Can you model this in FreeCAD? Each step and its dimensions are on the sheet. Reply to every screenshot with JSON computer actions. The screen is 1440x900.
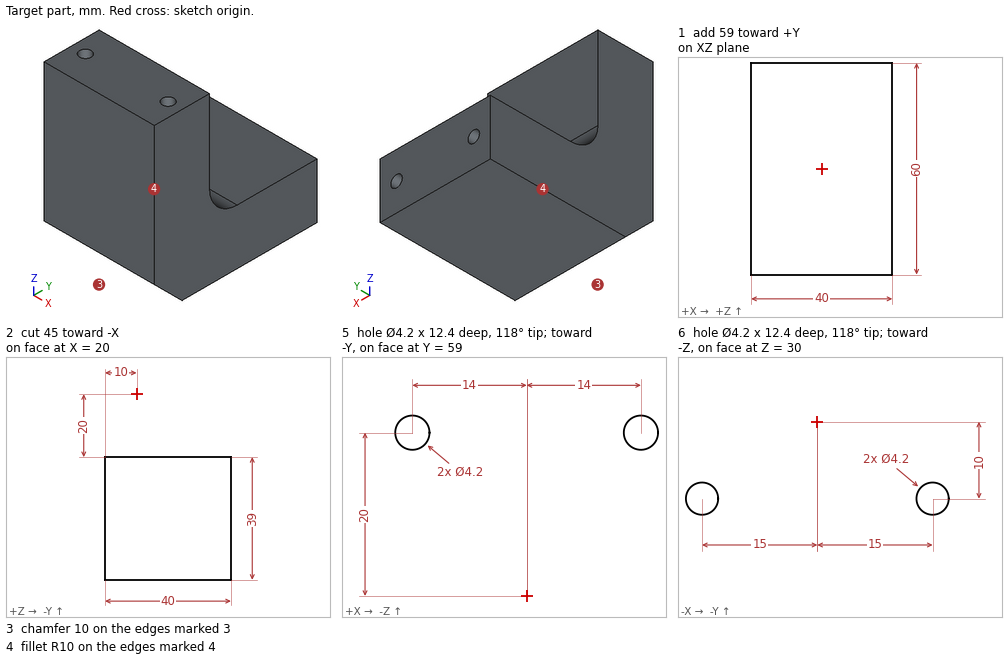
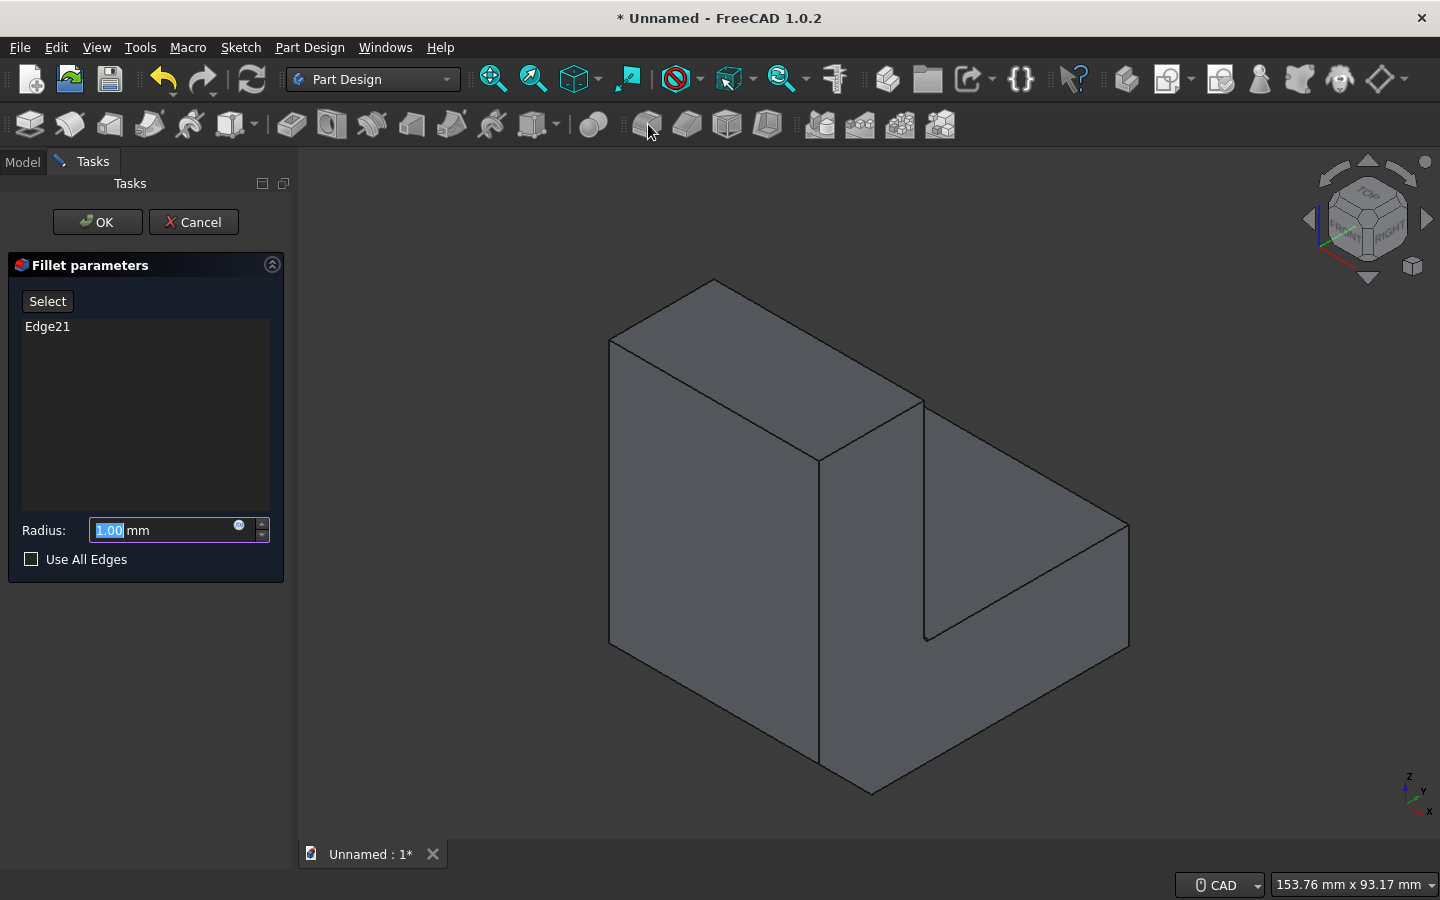
{"action": "type", "text": "10"}
{"action": "key", "text": "Tab"}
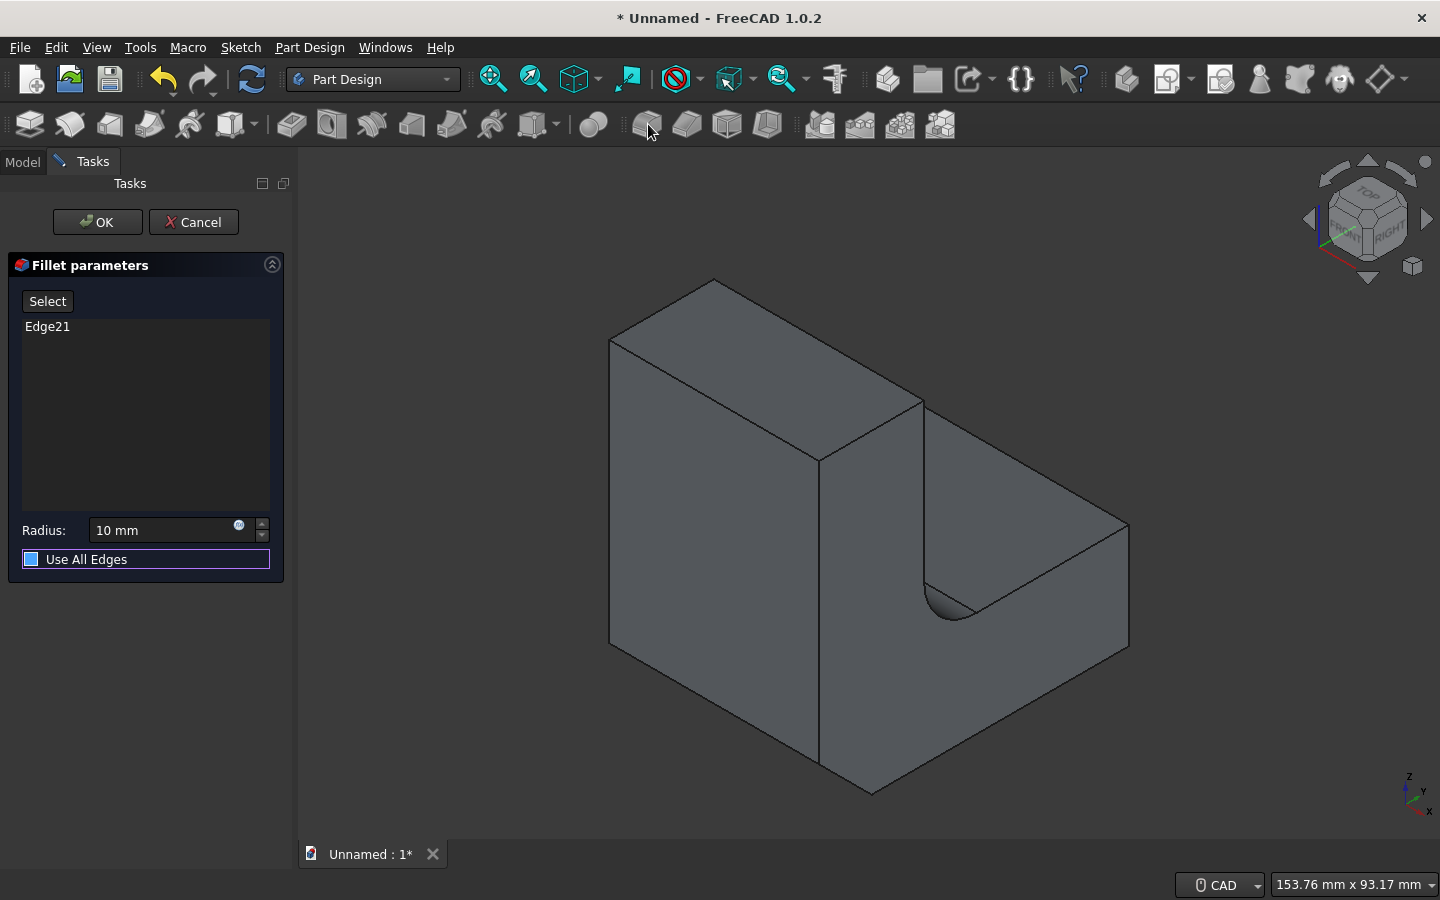
{"action": "left_click", "coordinate": [98, 222]}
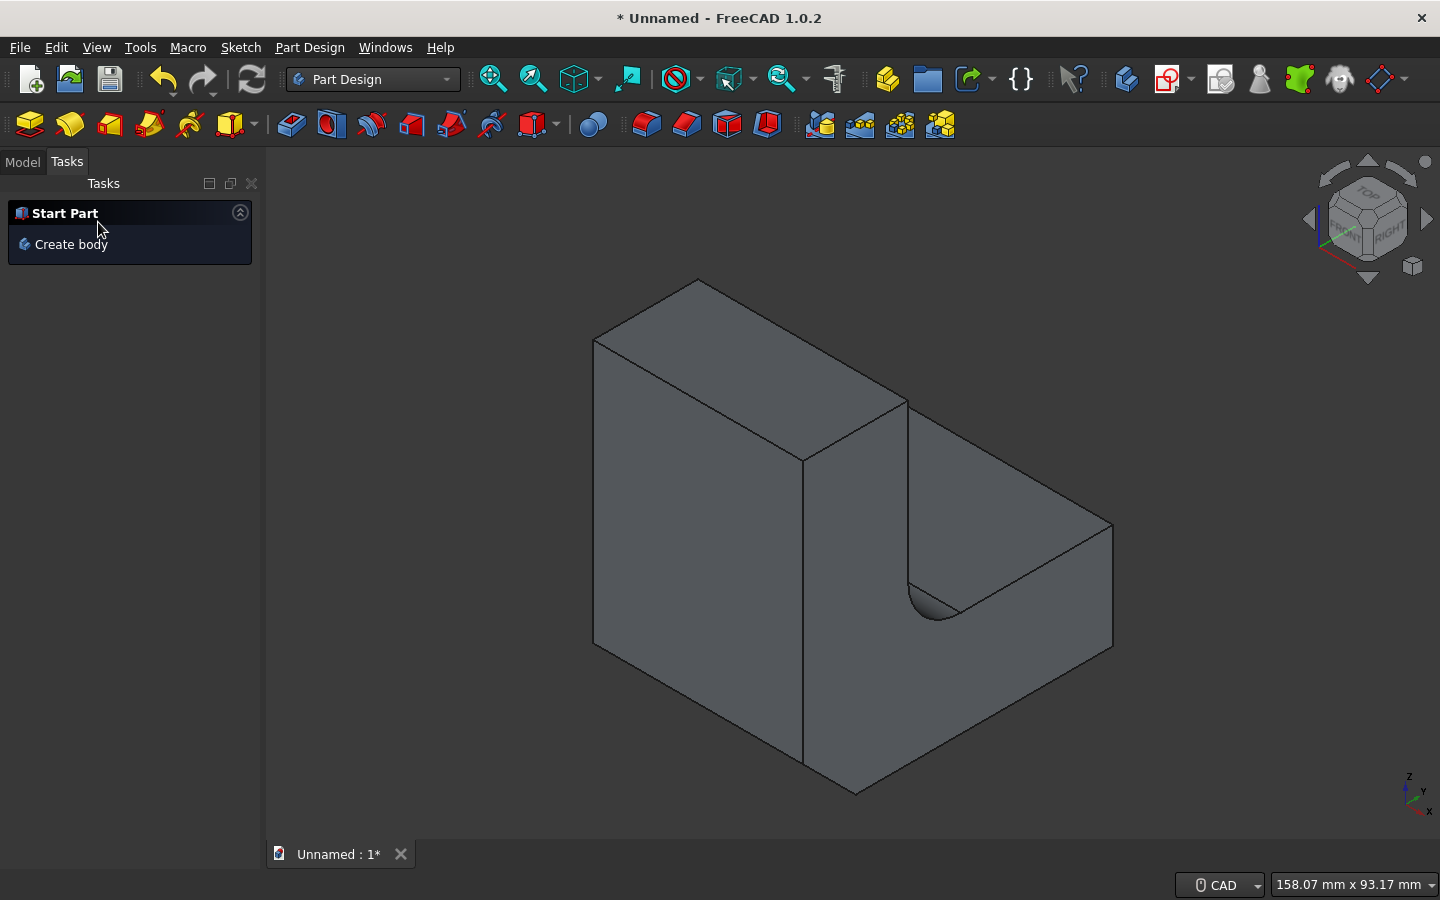
{"action": "key", "text": "4"}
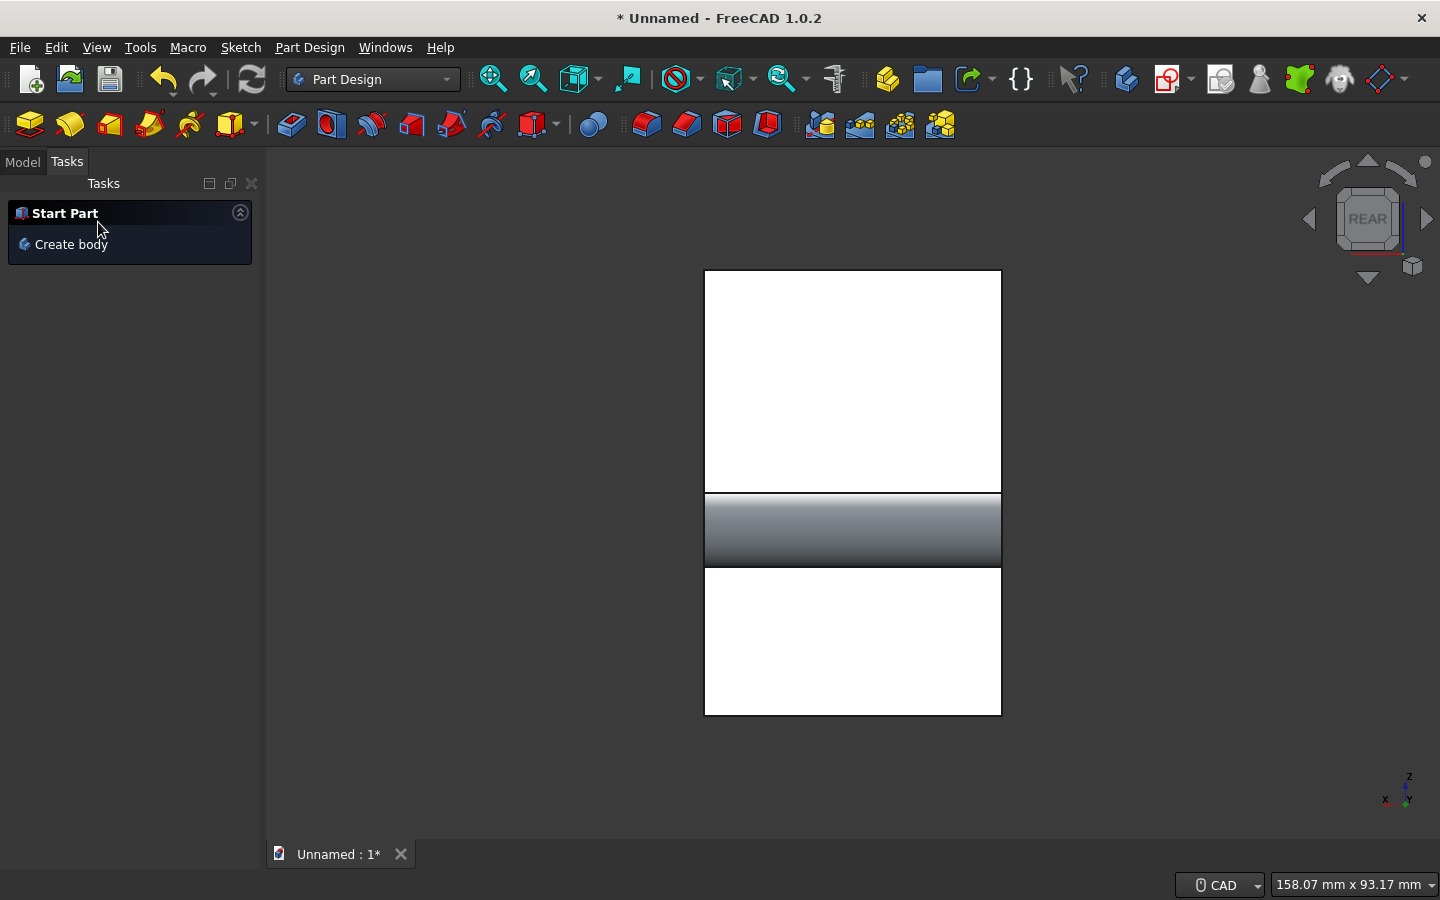
{"action": "left_click", "coordinate": [853, 641]}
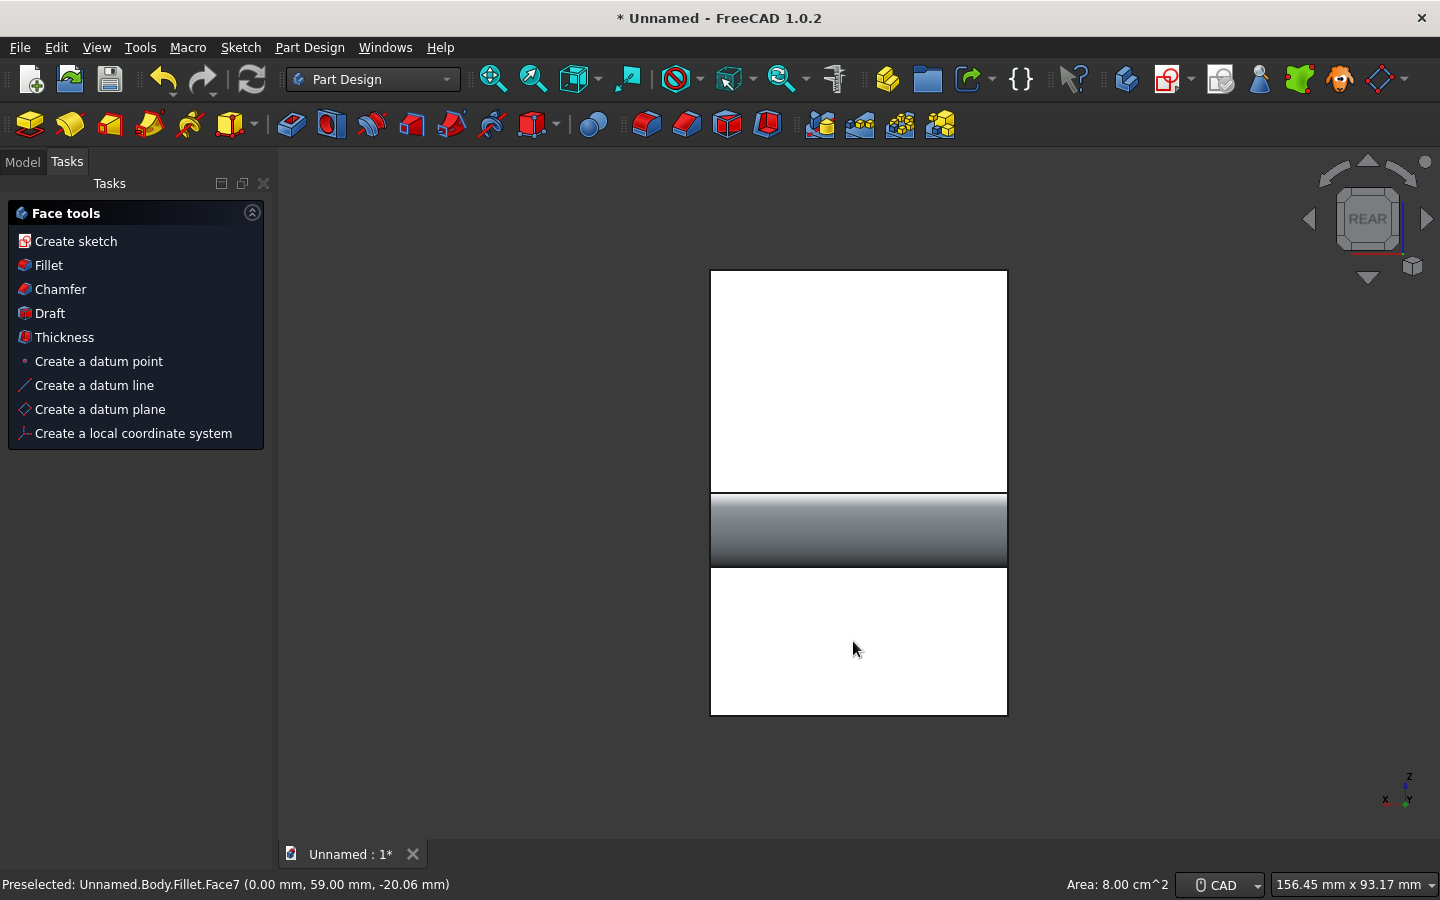
{"action": "left_click", "coordinate": [1168, 80]}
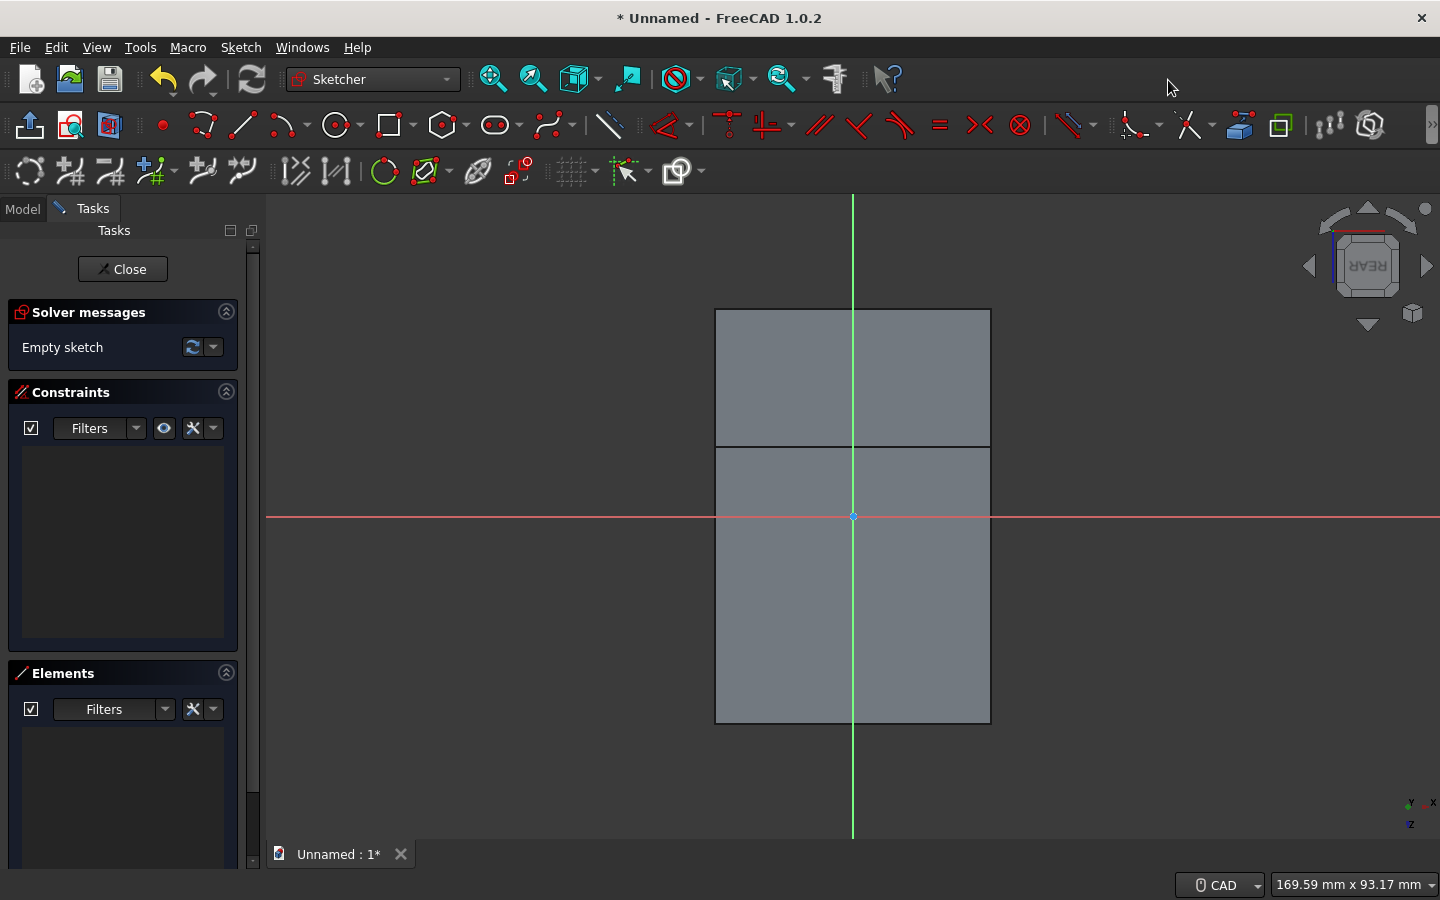
{"action": "scroll", "coordinate": [893, 395], "scroll_direction": "up", "scroll_amount": 5}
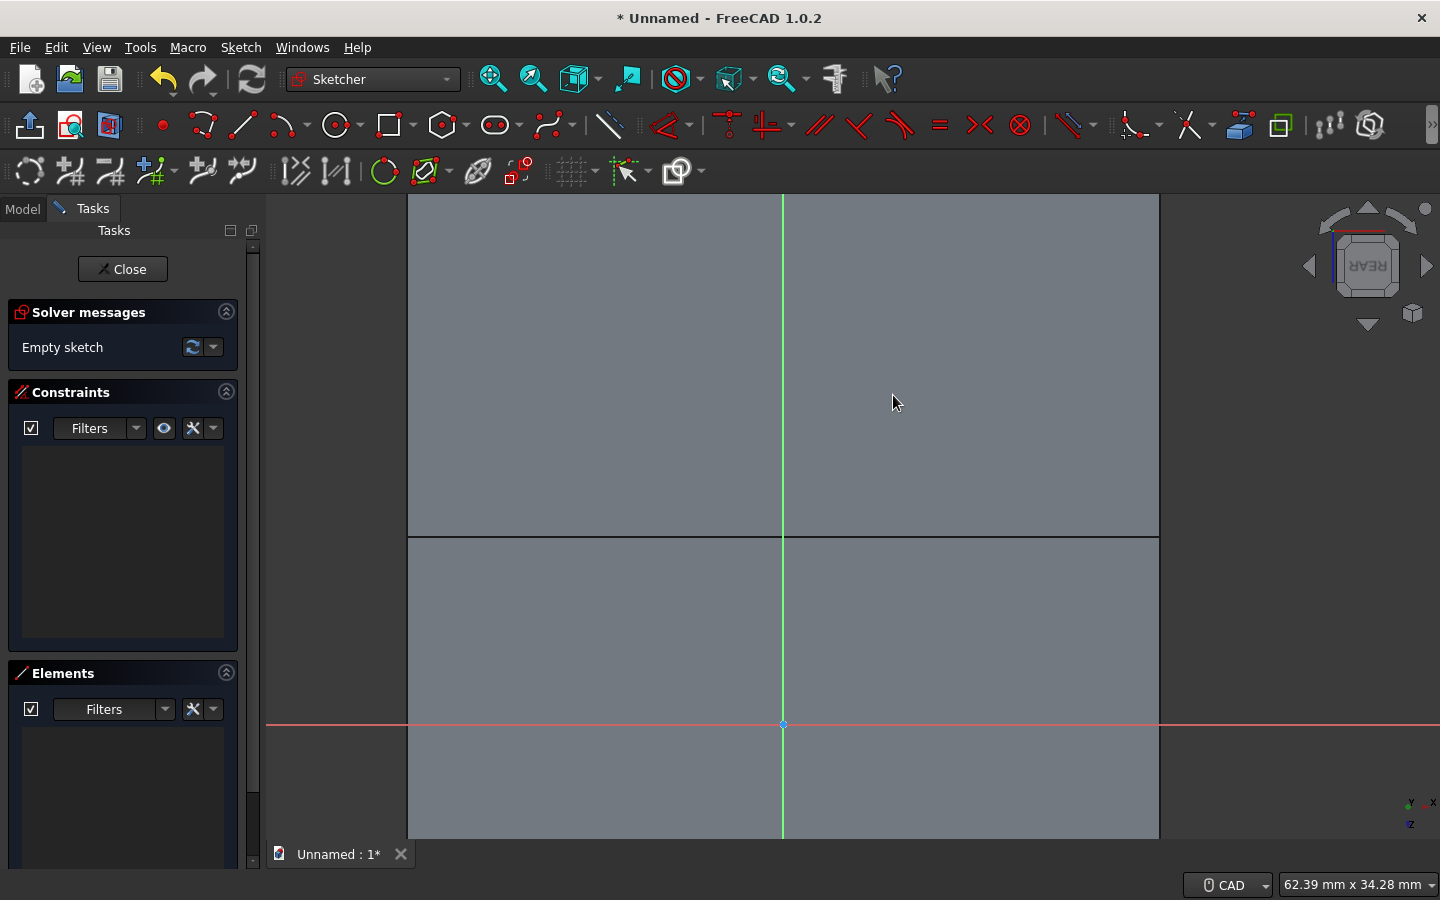
{"action": "left_click", "coordinate": [336, 126]}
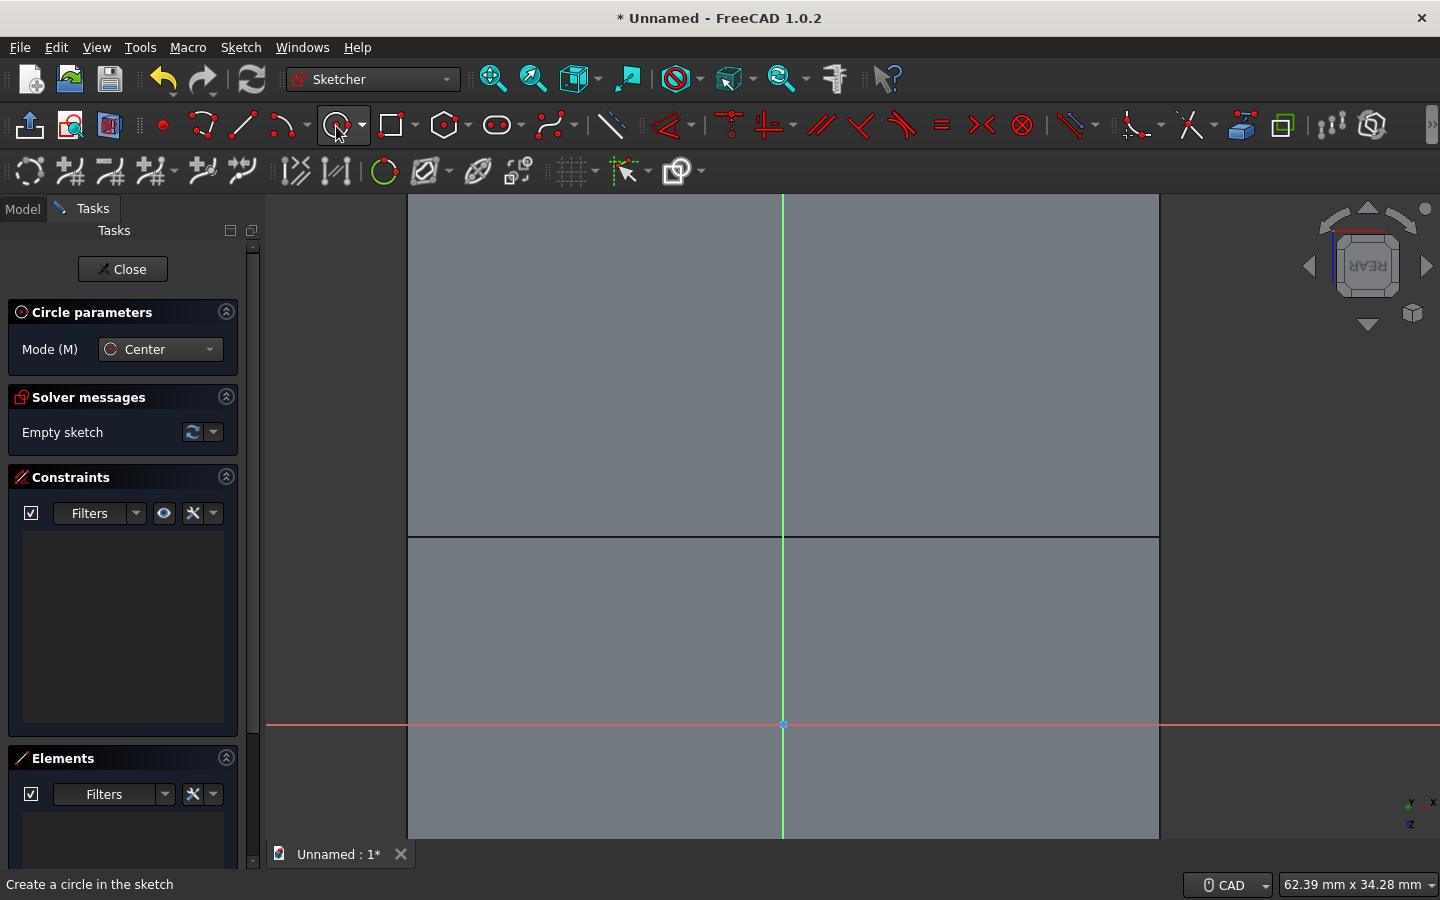
{"action": "left_click", "coordinate": [520, 348]}
{"action": "mouse_move", "coordinate": [548, 320]}